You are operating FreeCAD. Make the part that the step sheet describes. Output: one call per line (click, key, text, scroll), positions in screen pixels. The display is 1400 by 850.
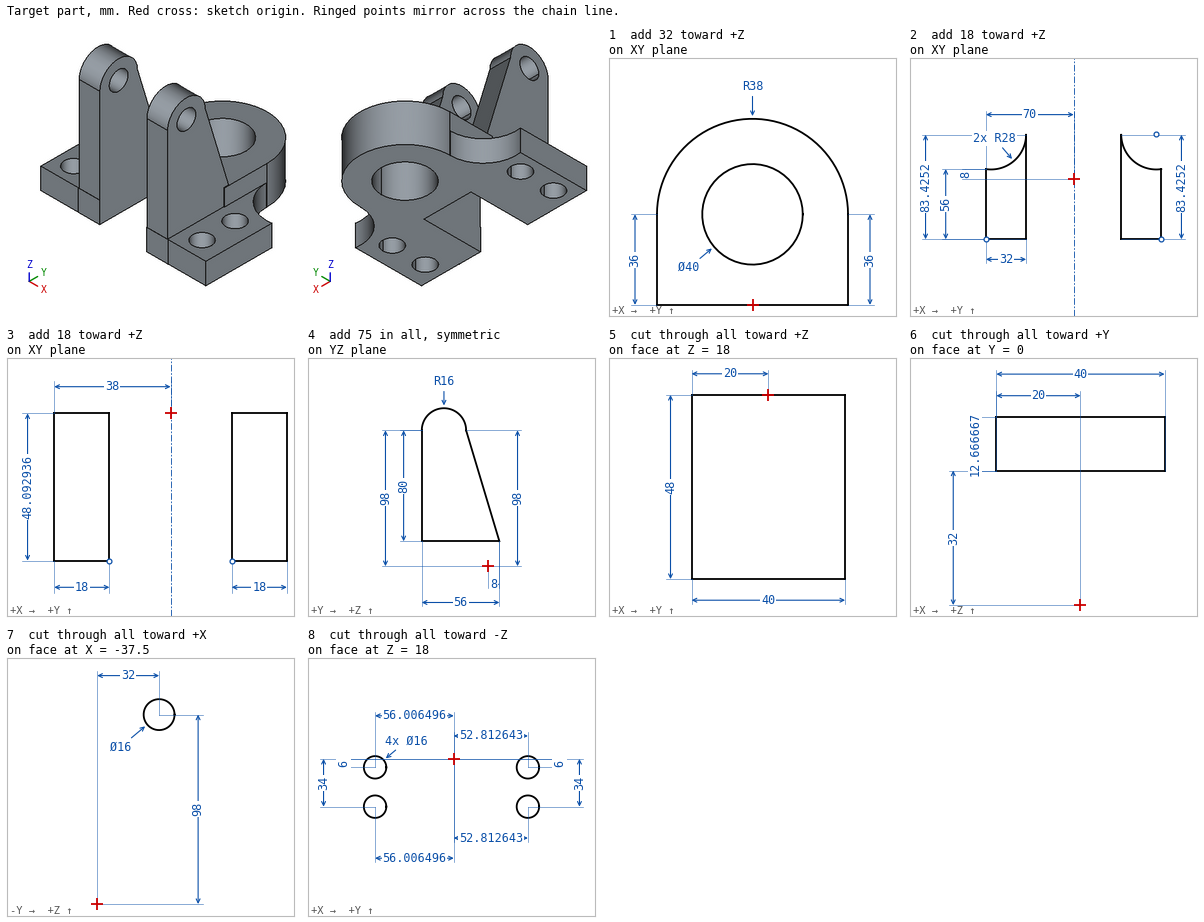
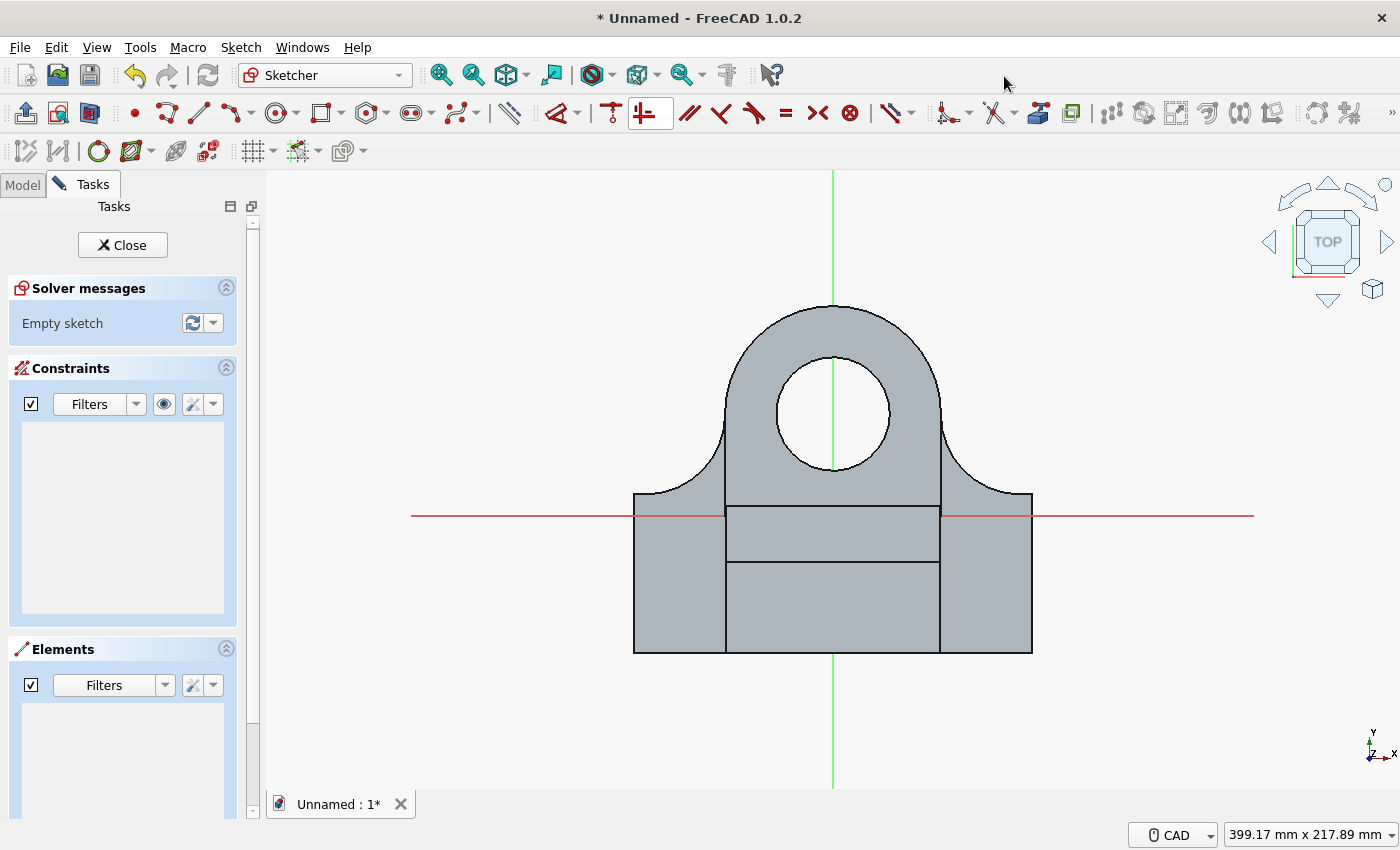
click(90, 114)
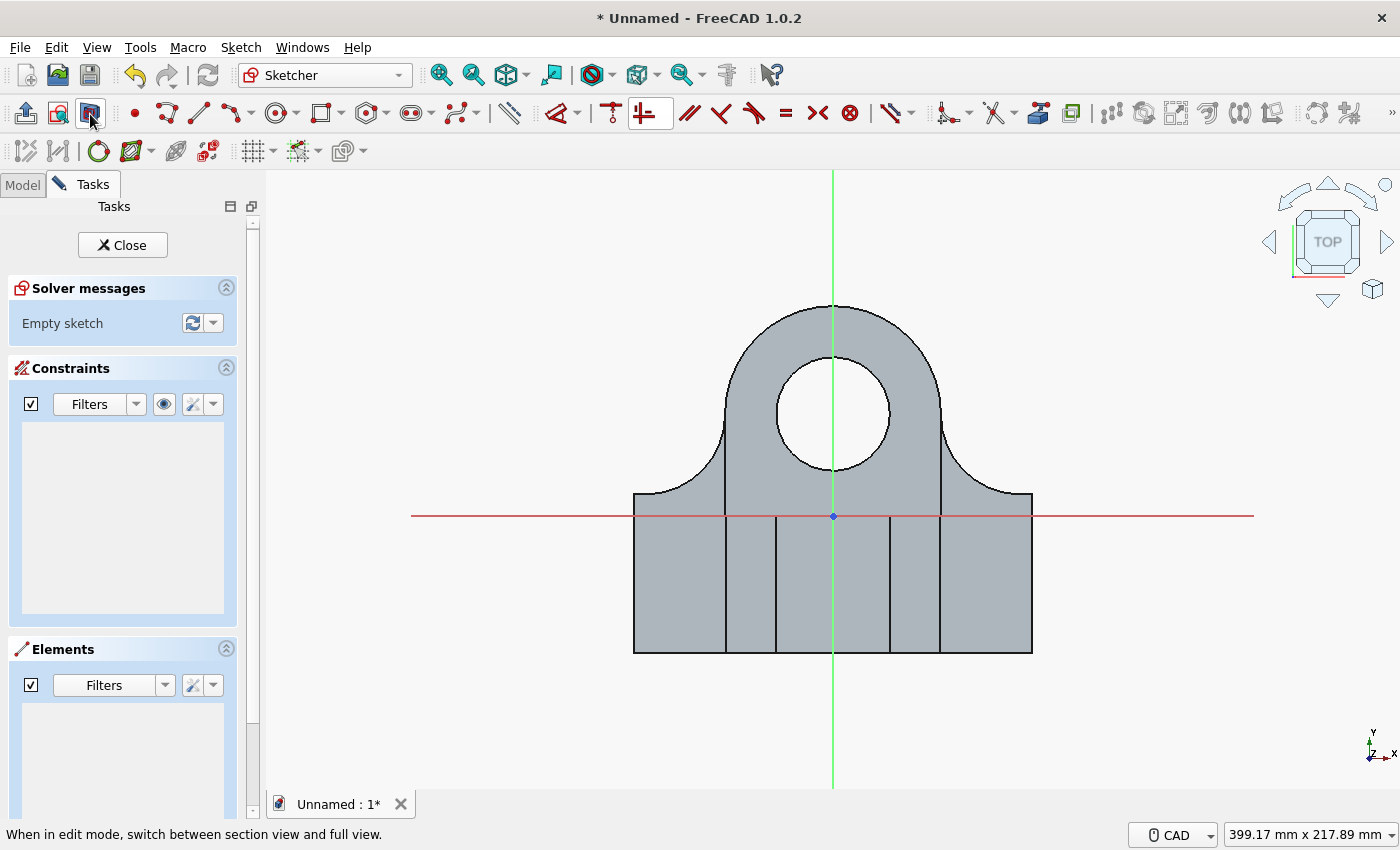
scroll(873, 646, up, 5)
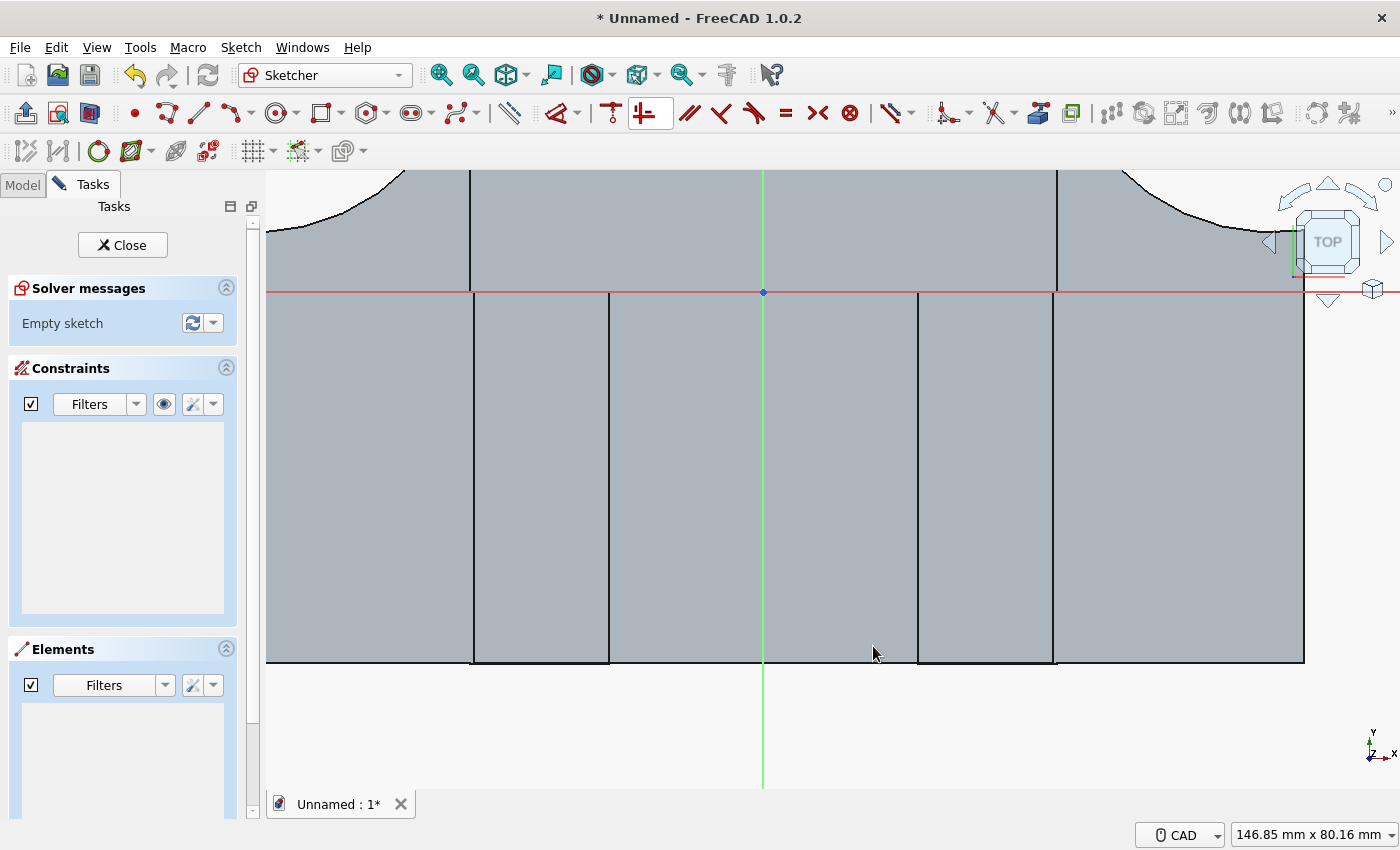
click(322, 114)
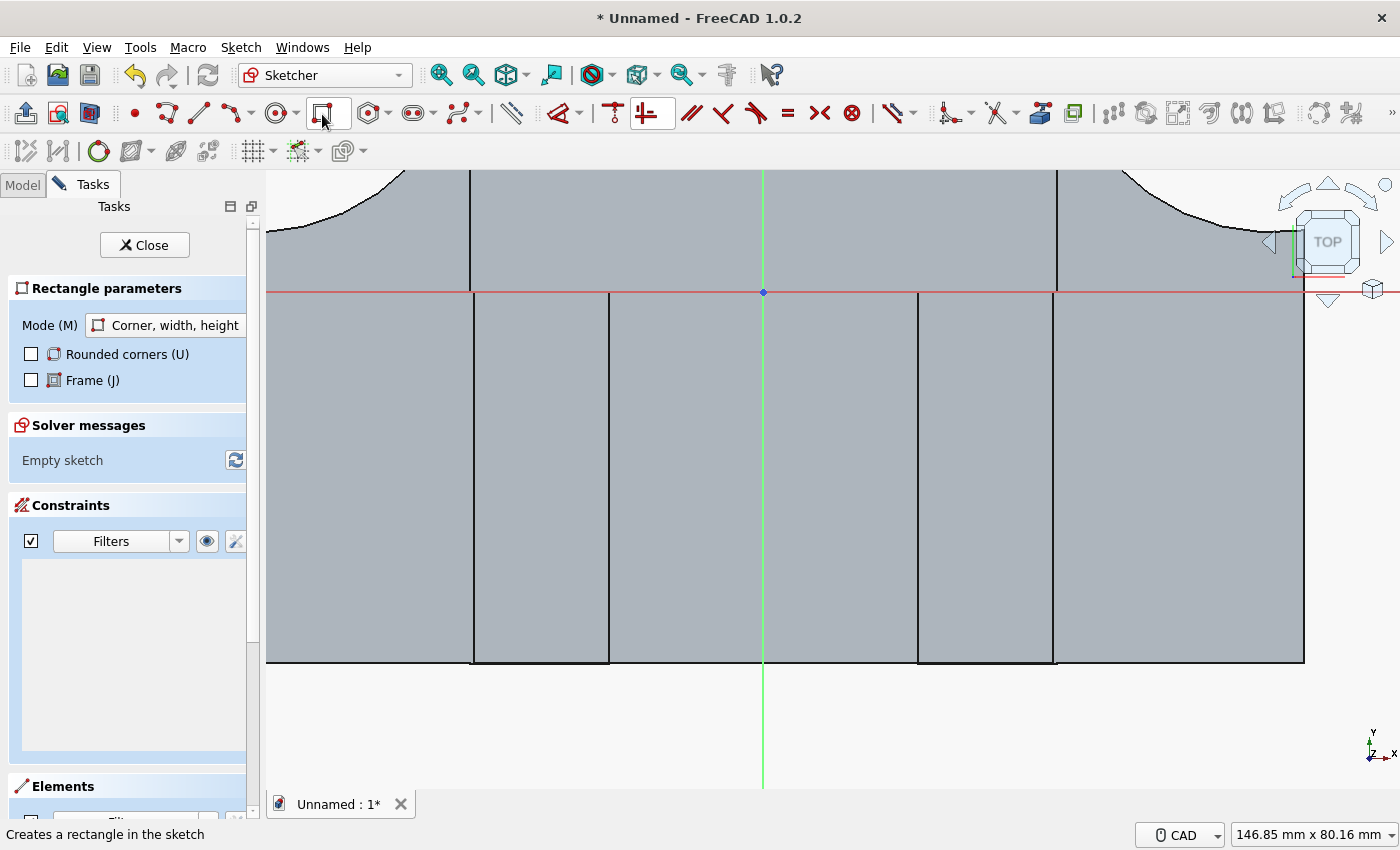
click(609, 292)
click(918, 663)
key(Escape)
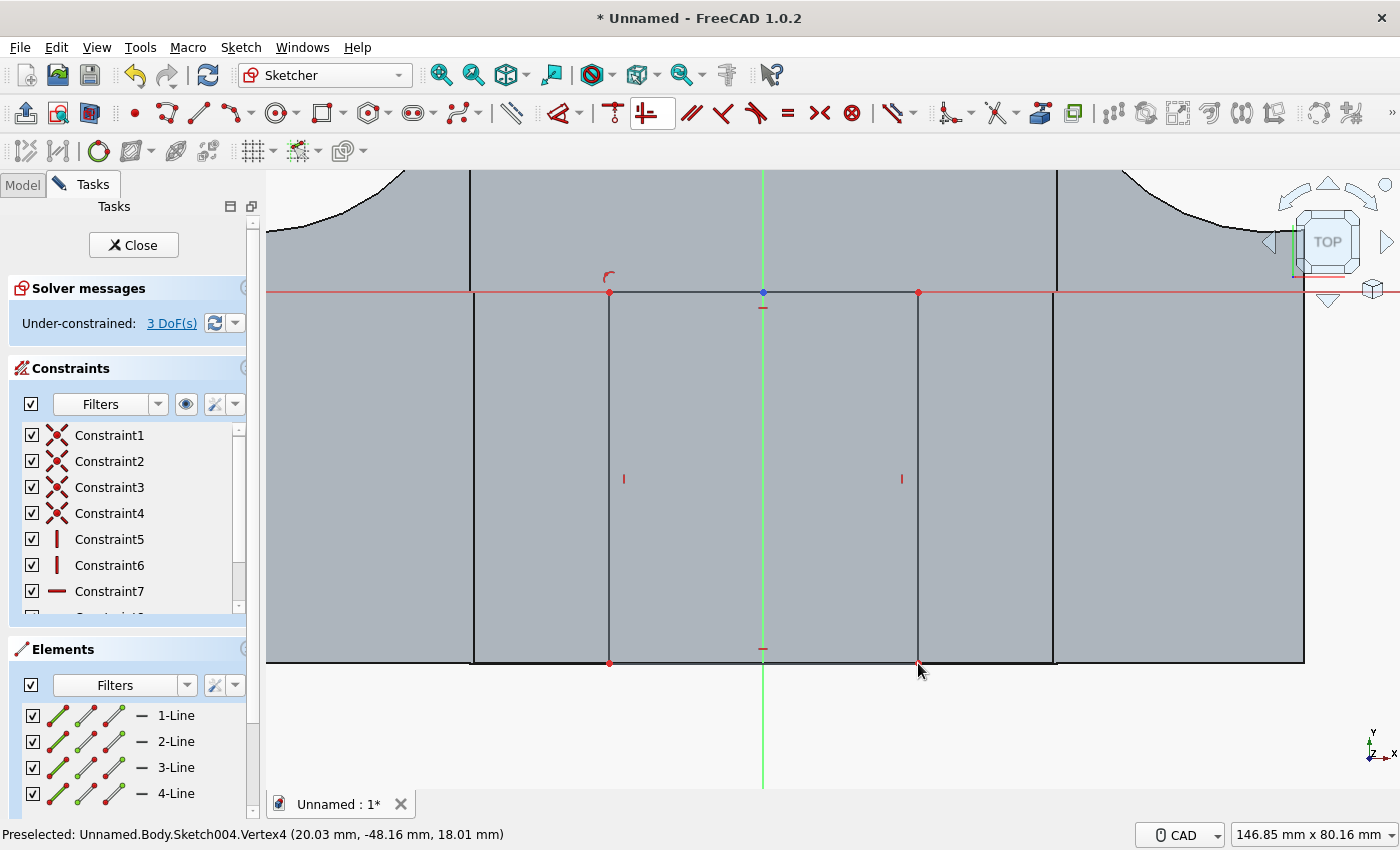
click(558, 114)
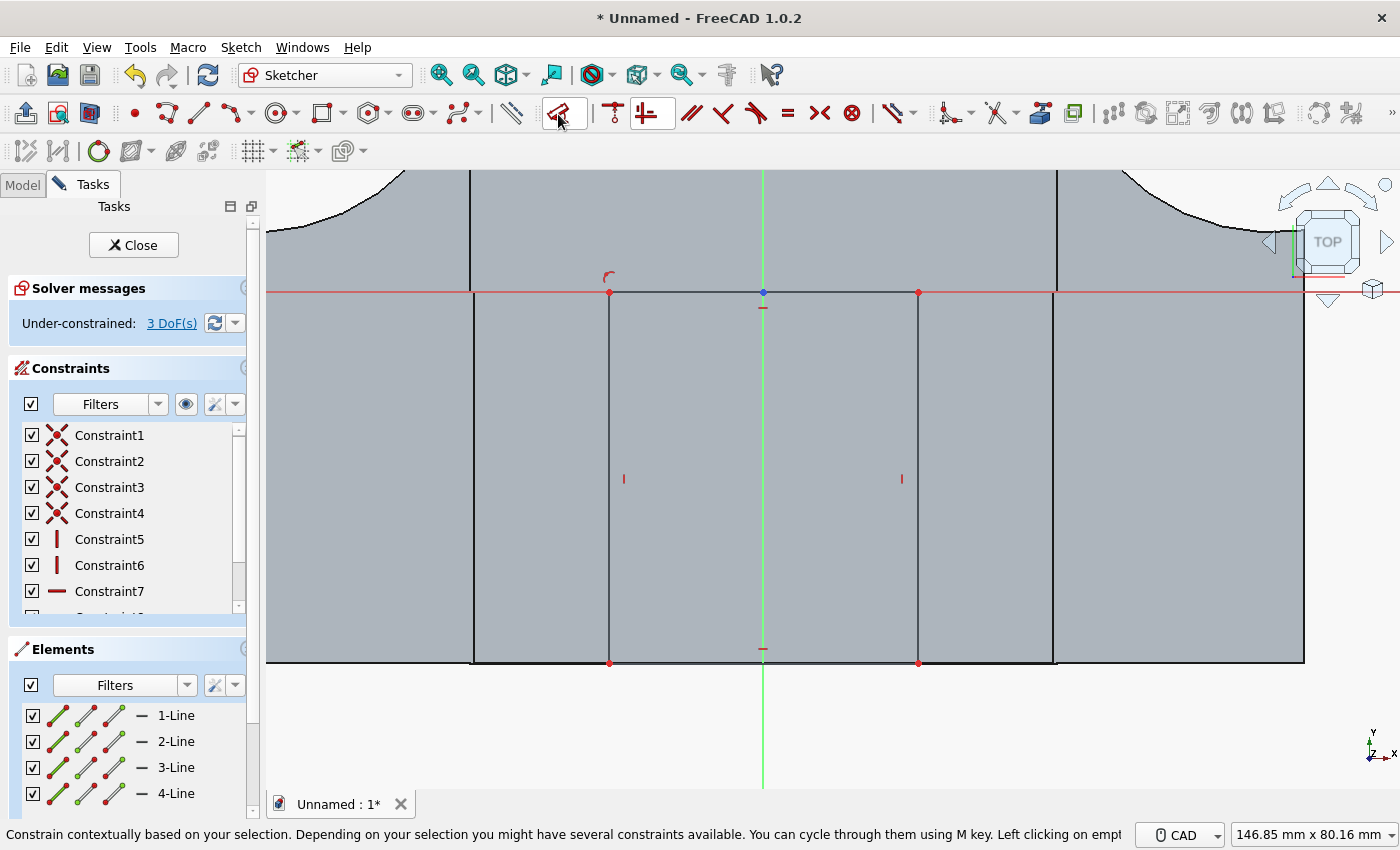
click(609, 404)
click(575, 478)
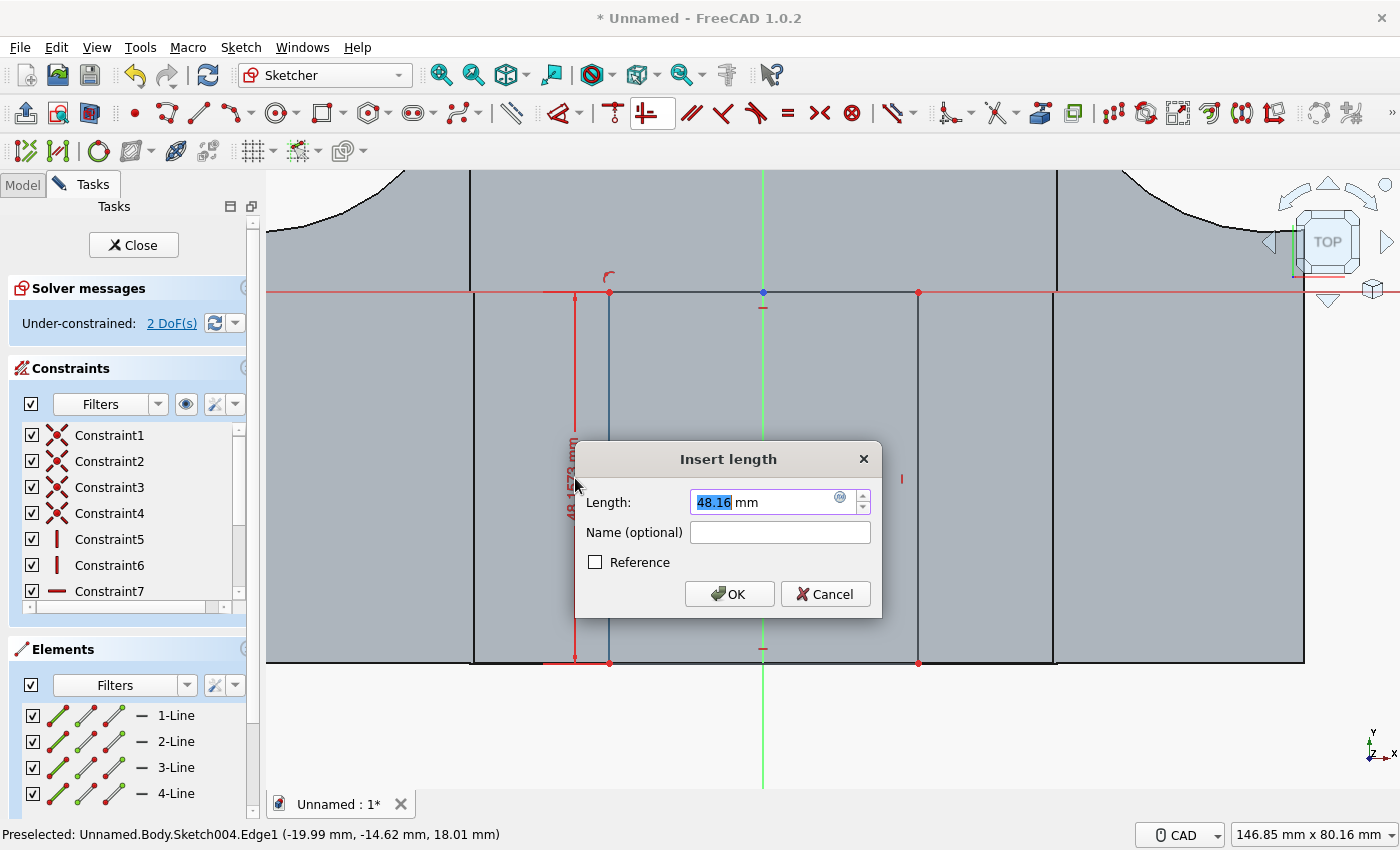
text(48)
key(Return)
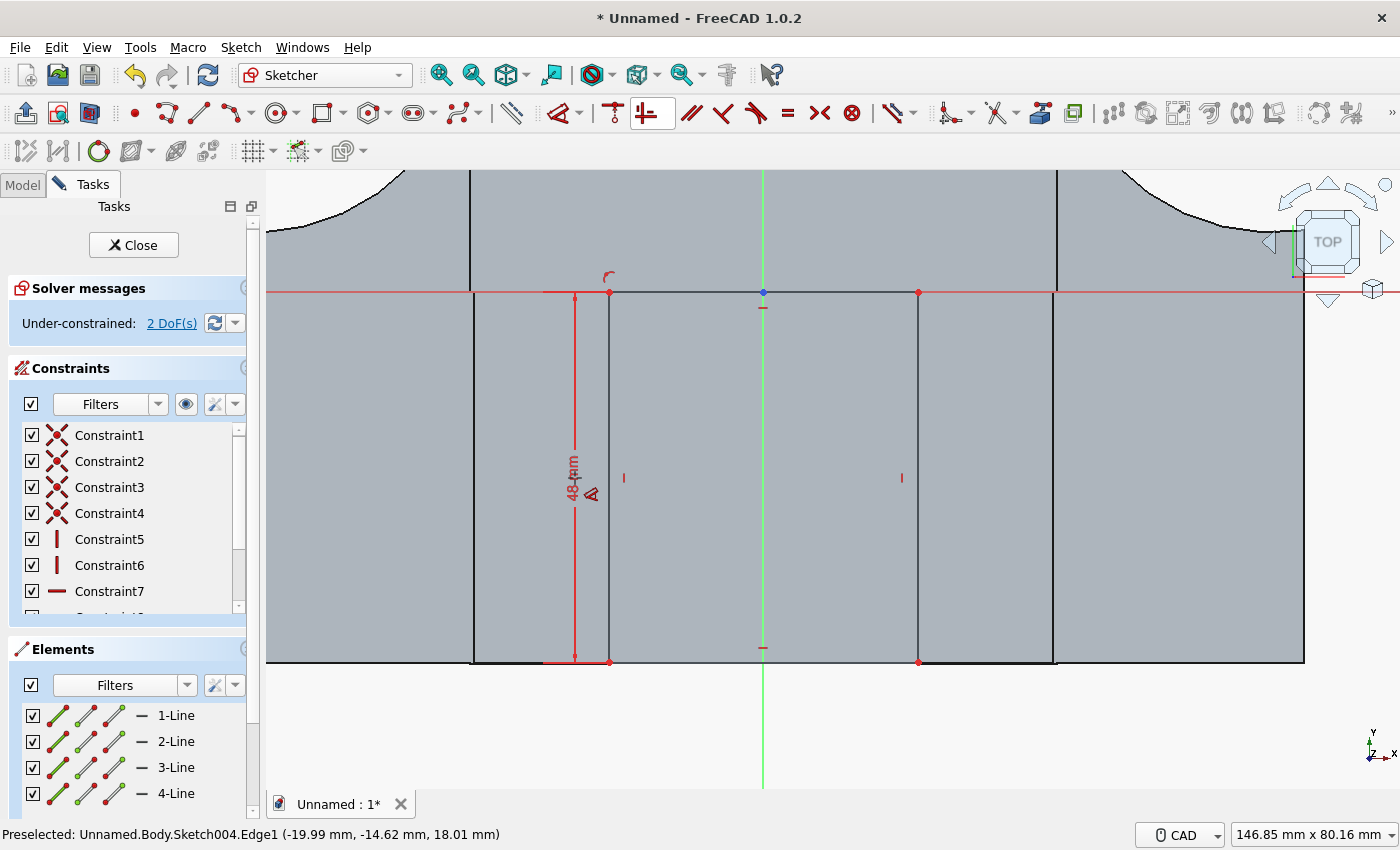
click(702, 663)
click(692, 697)